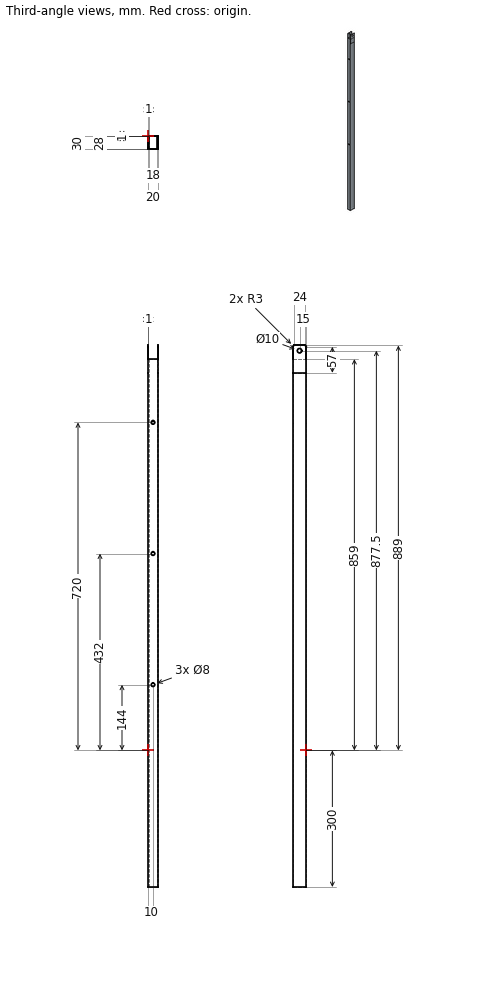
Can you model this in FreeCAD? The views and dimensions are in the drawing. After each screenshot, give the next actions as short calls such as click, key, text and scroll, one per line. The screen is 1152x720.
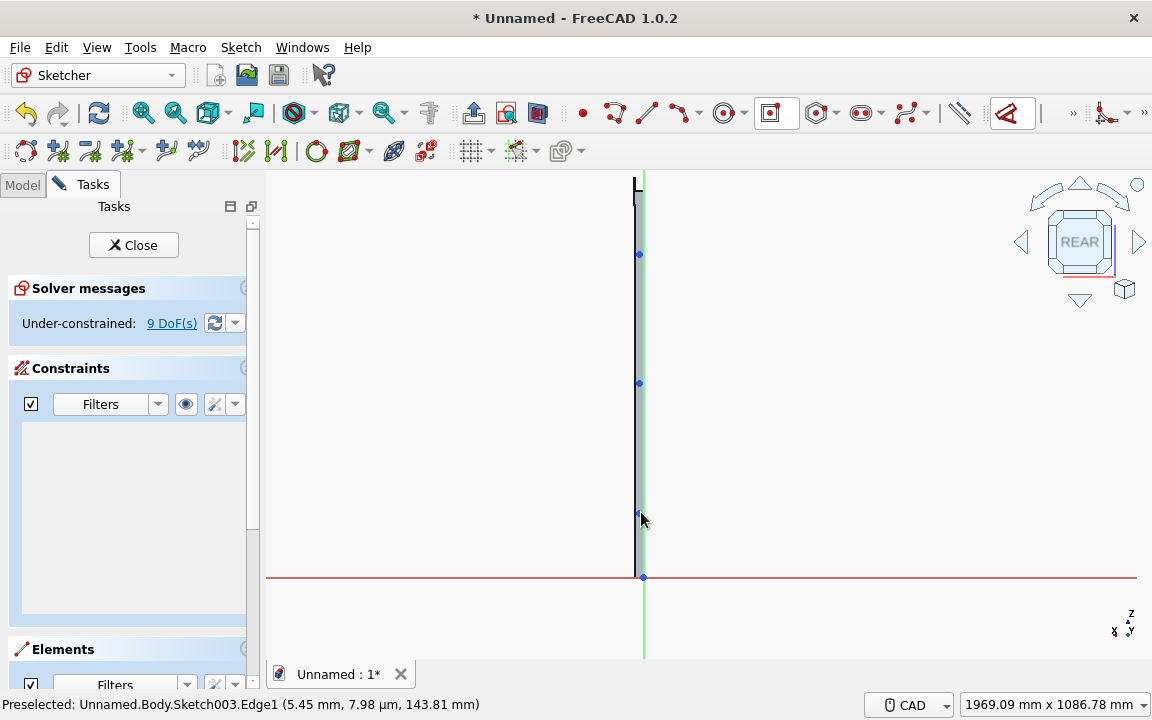
scroll(640, 382, up, 11)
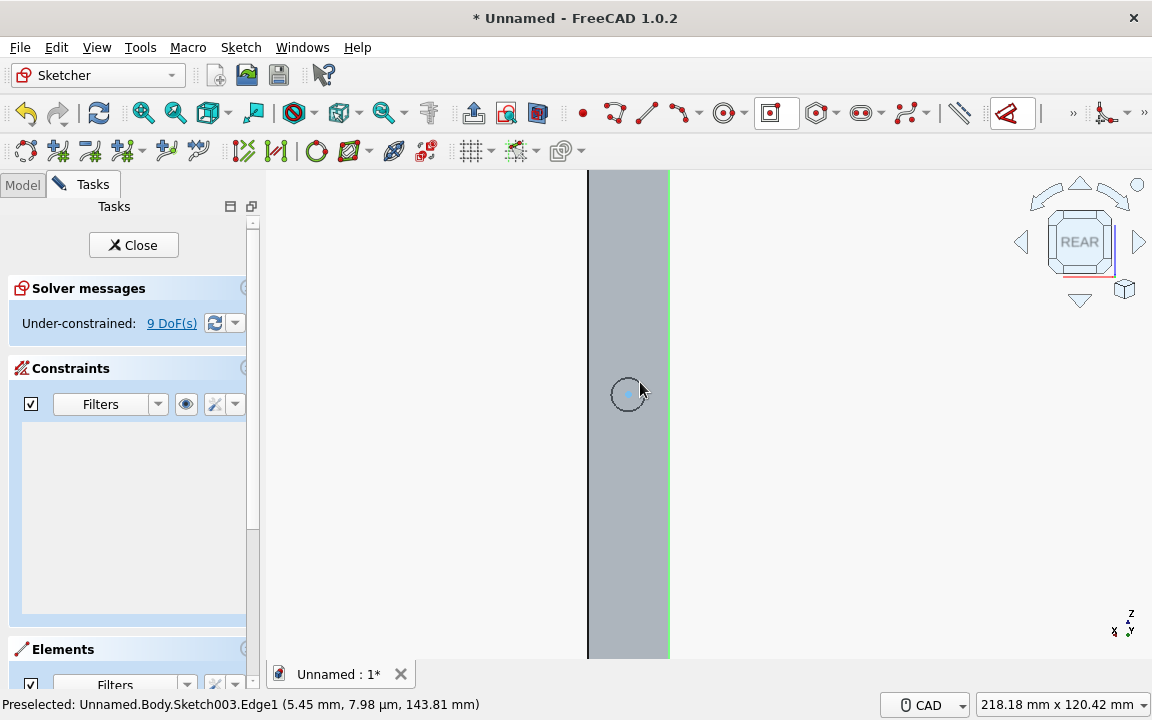
click(640, 383)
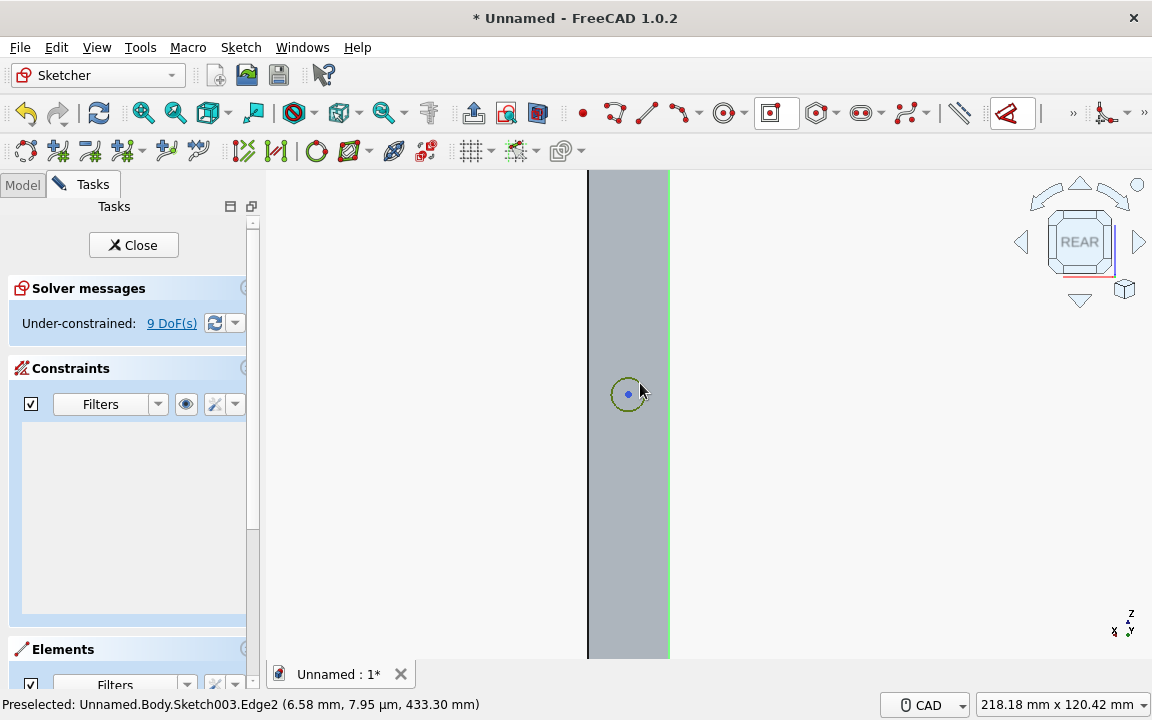
scroll(640, 382, down, 11)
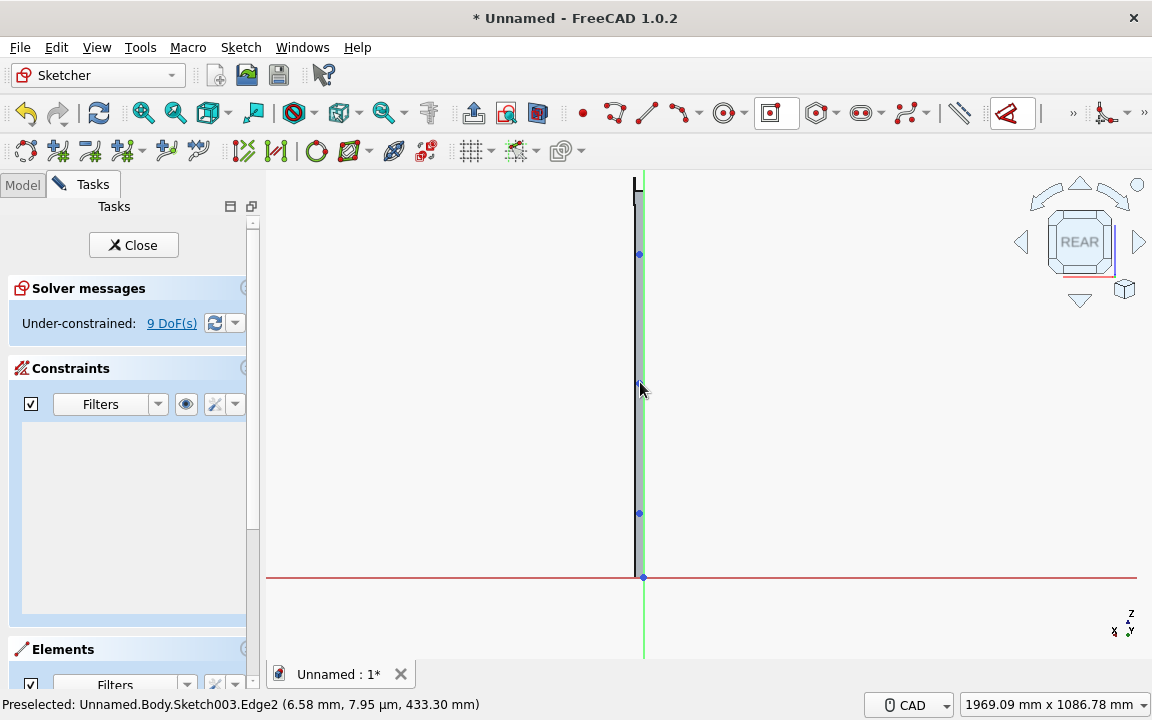
scroll(641, 253, up, 10)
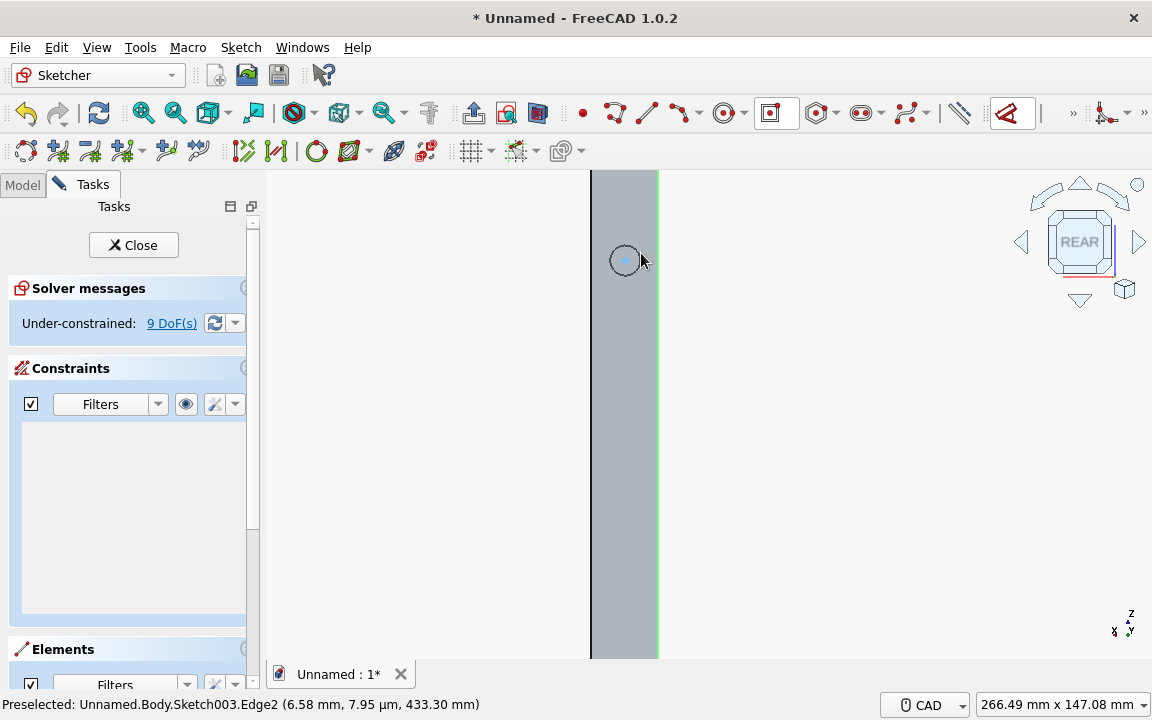
click(636, 250)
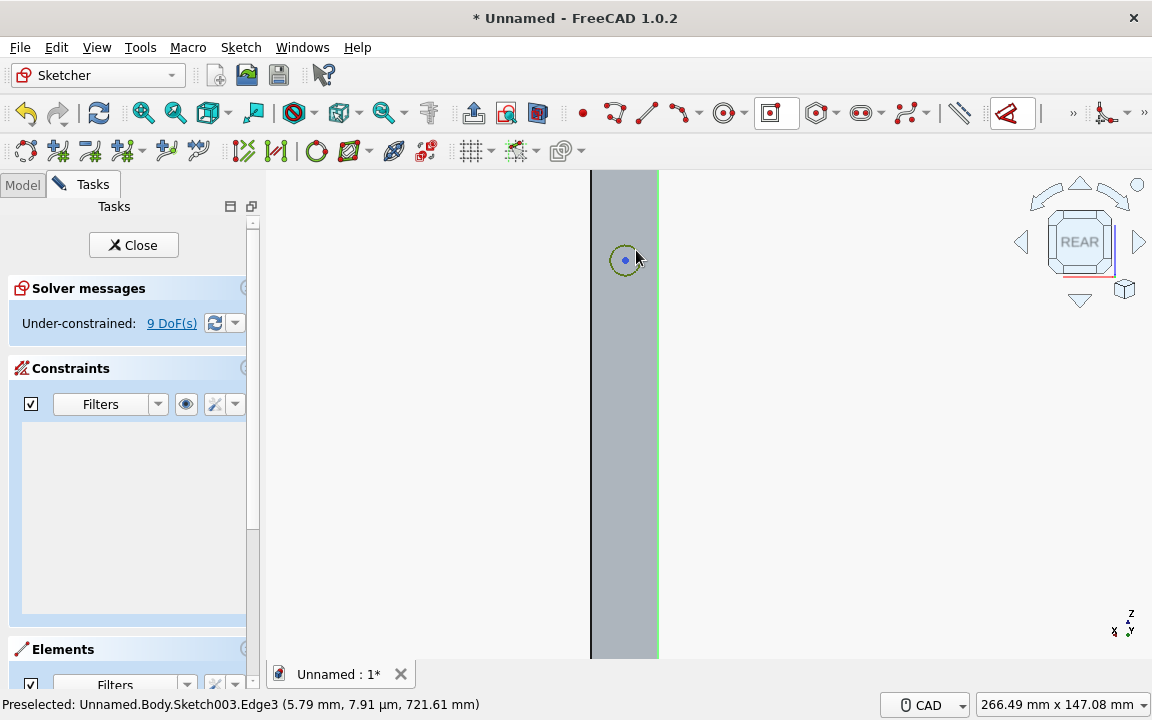
key(e)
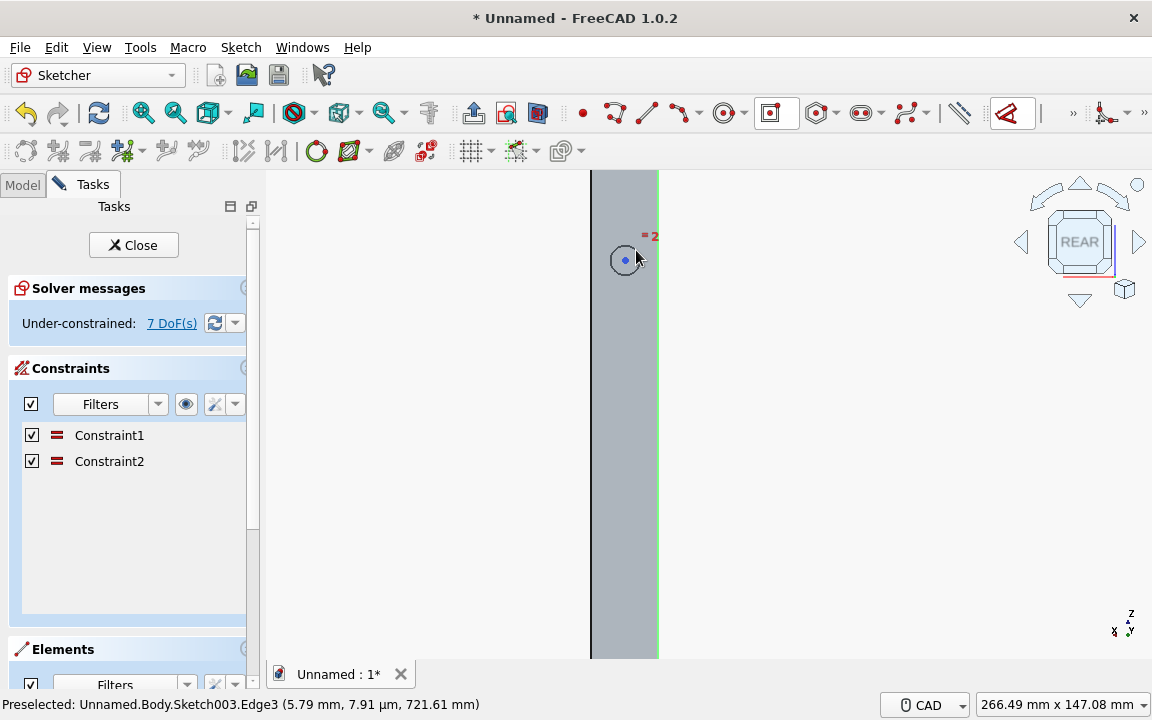
scroll(641, 253, down, 10)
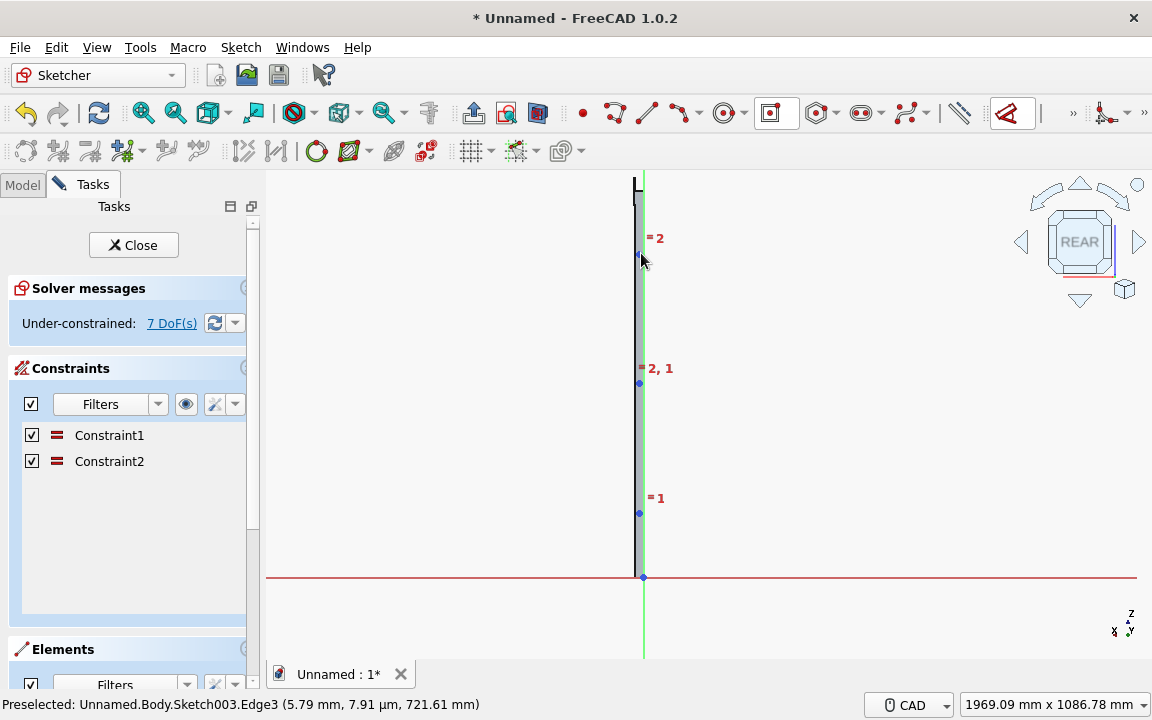
scroll(641, 512, up, 13)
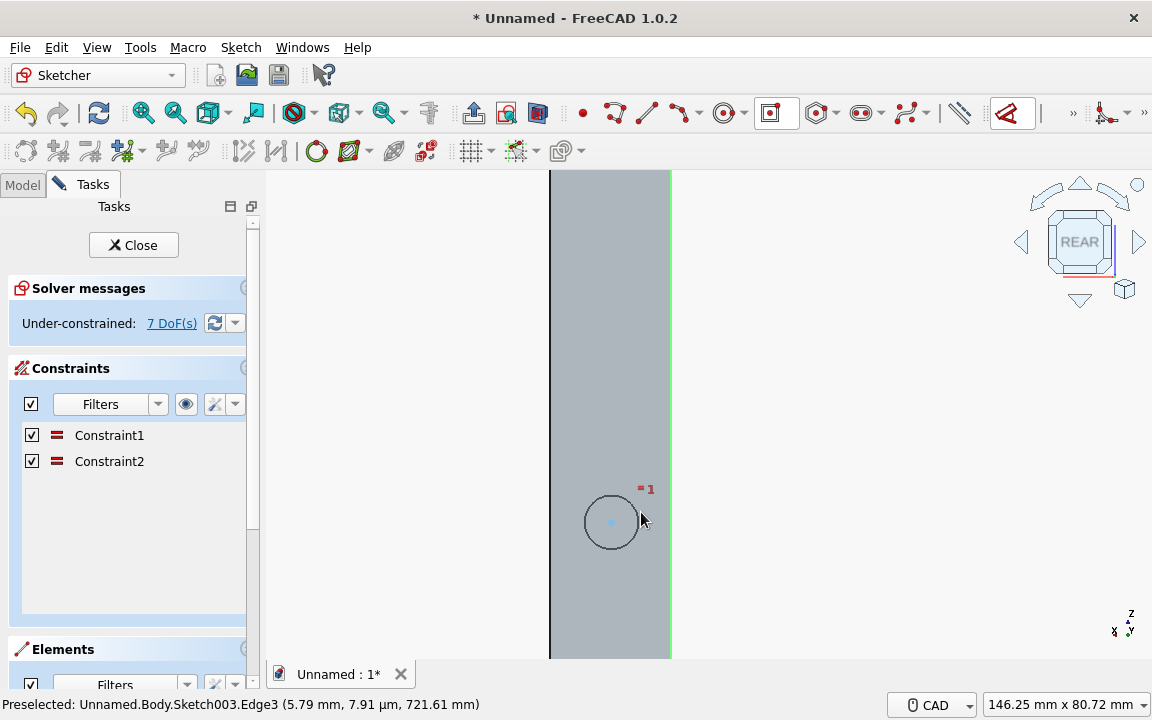
click(630, 503)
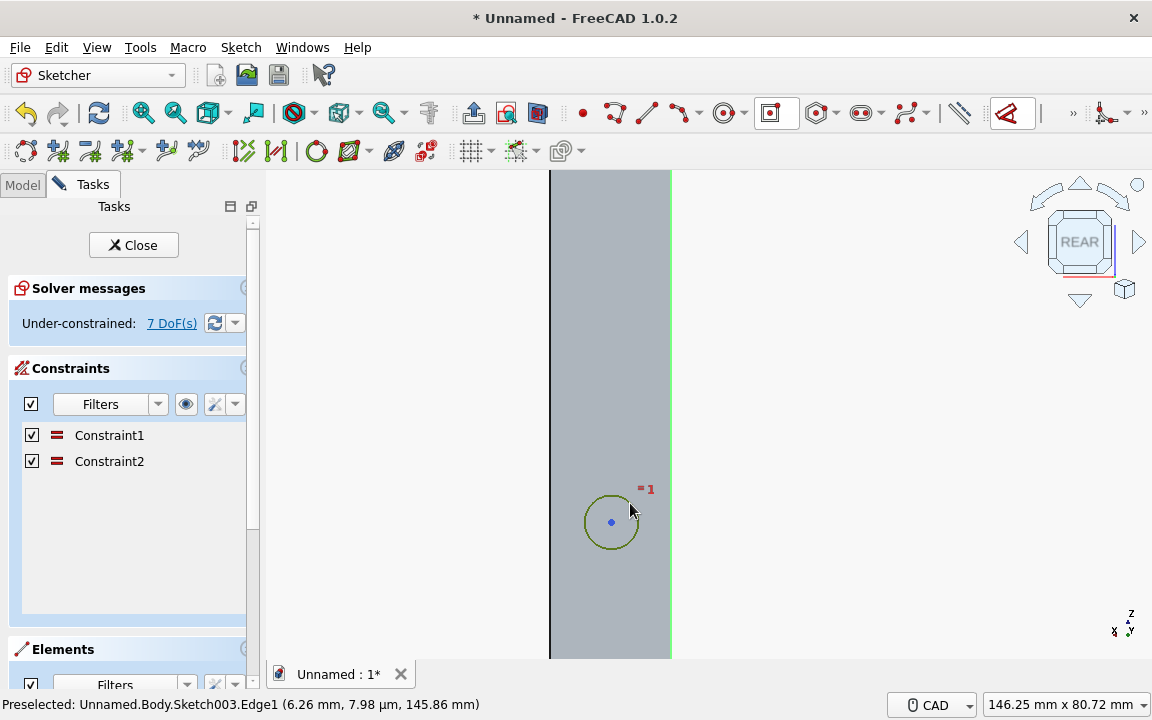
click(1030, 114)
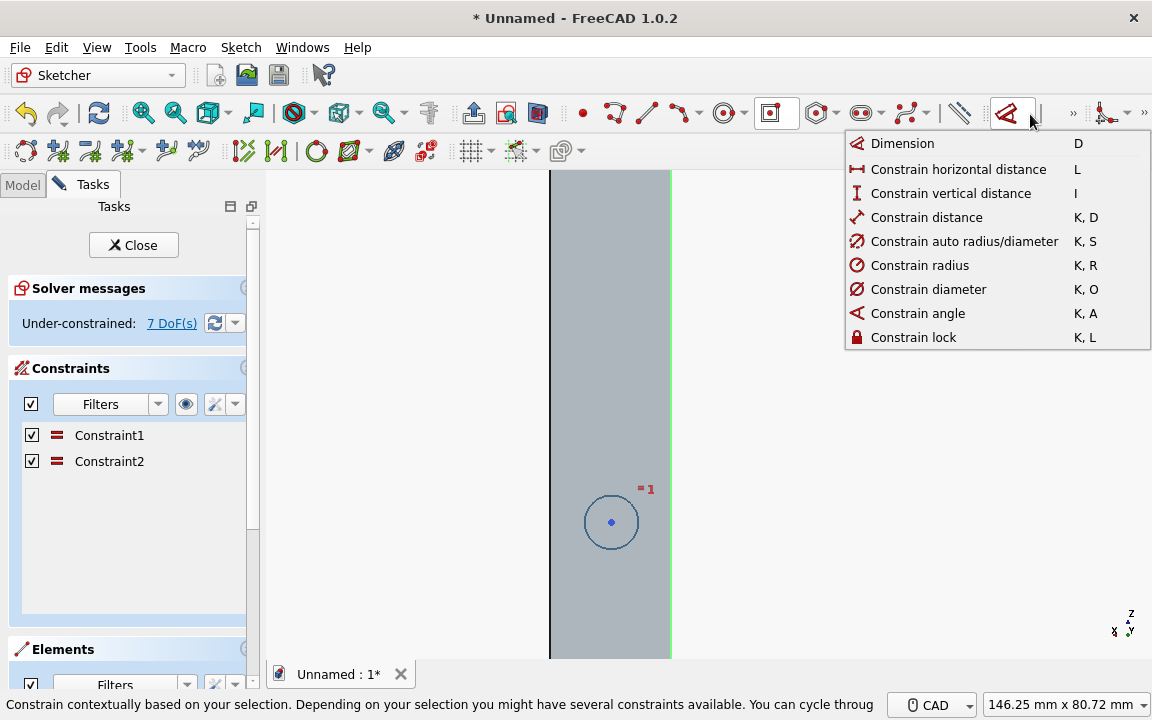
click(998, 289)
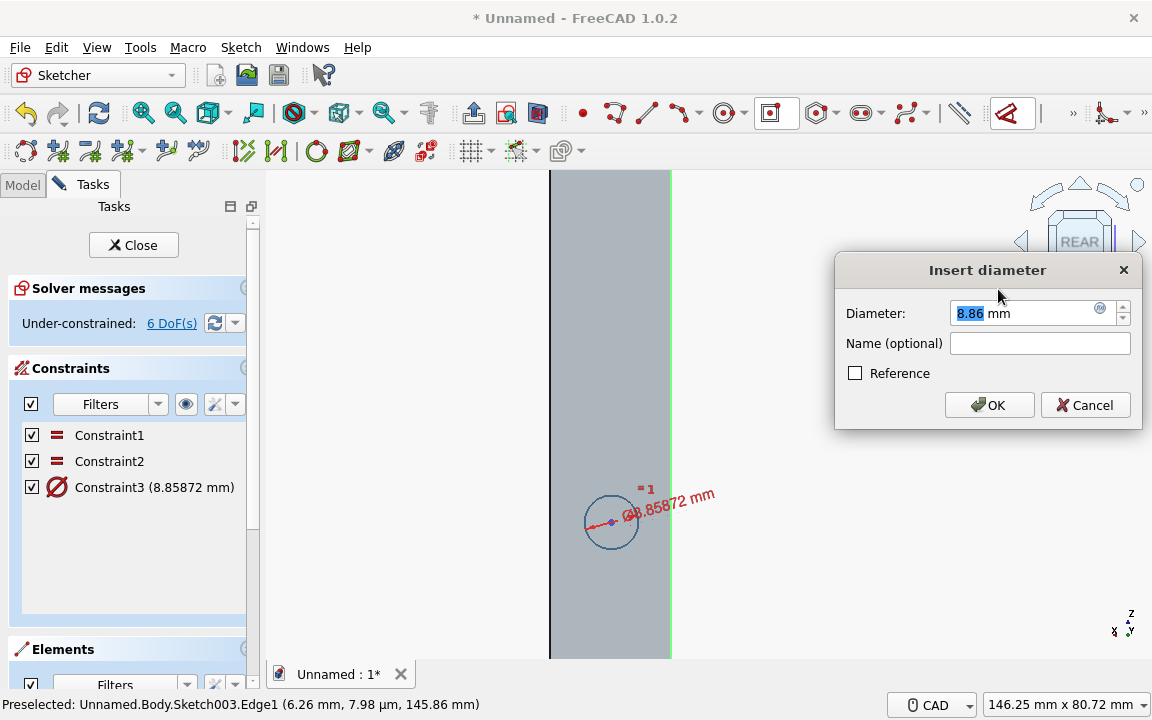
text(8)
key(Return)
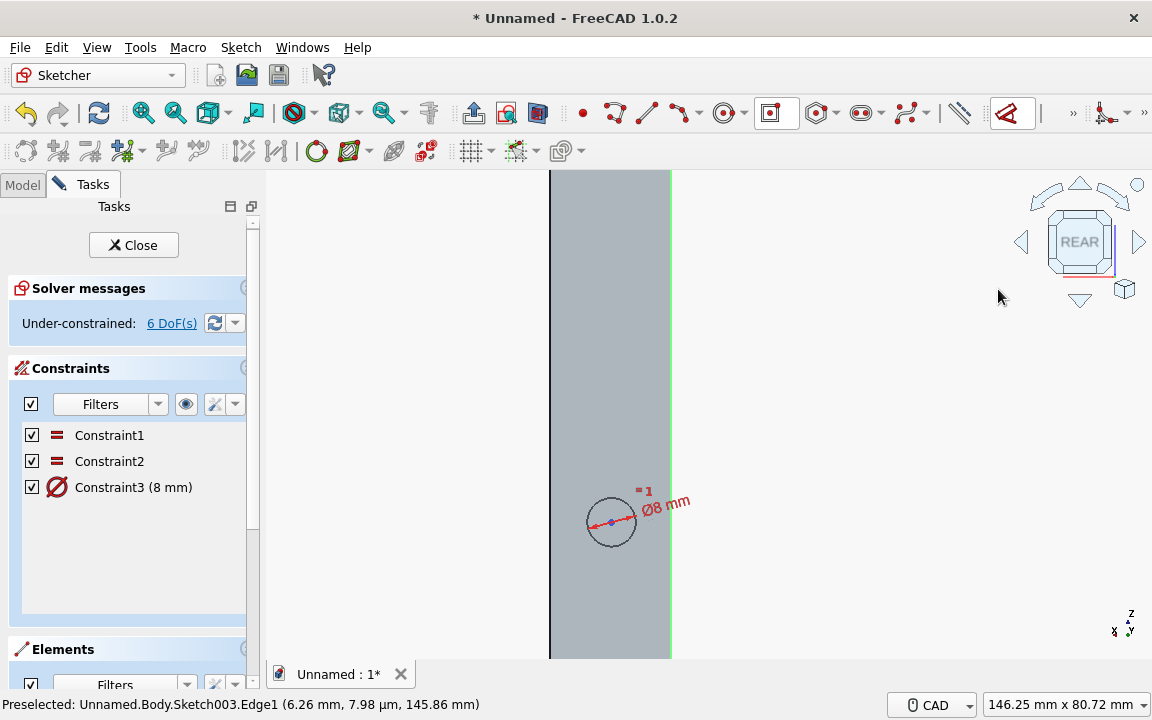
click(612, 522)